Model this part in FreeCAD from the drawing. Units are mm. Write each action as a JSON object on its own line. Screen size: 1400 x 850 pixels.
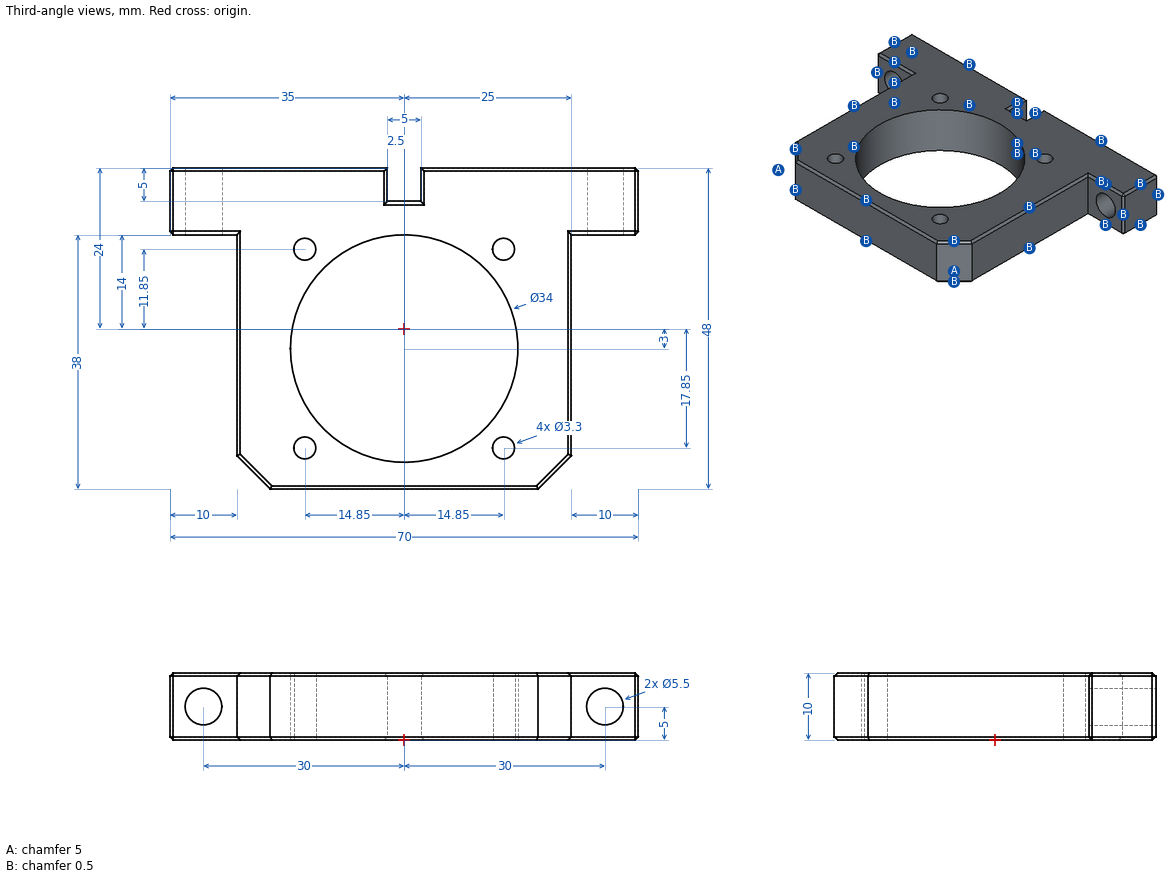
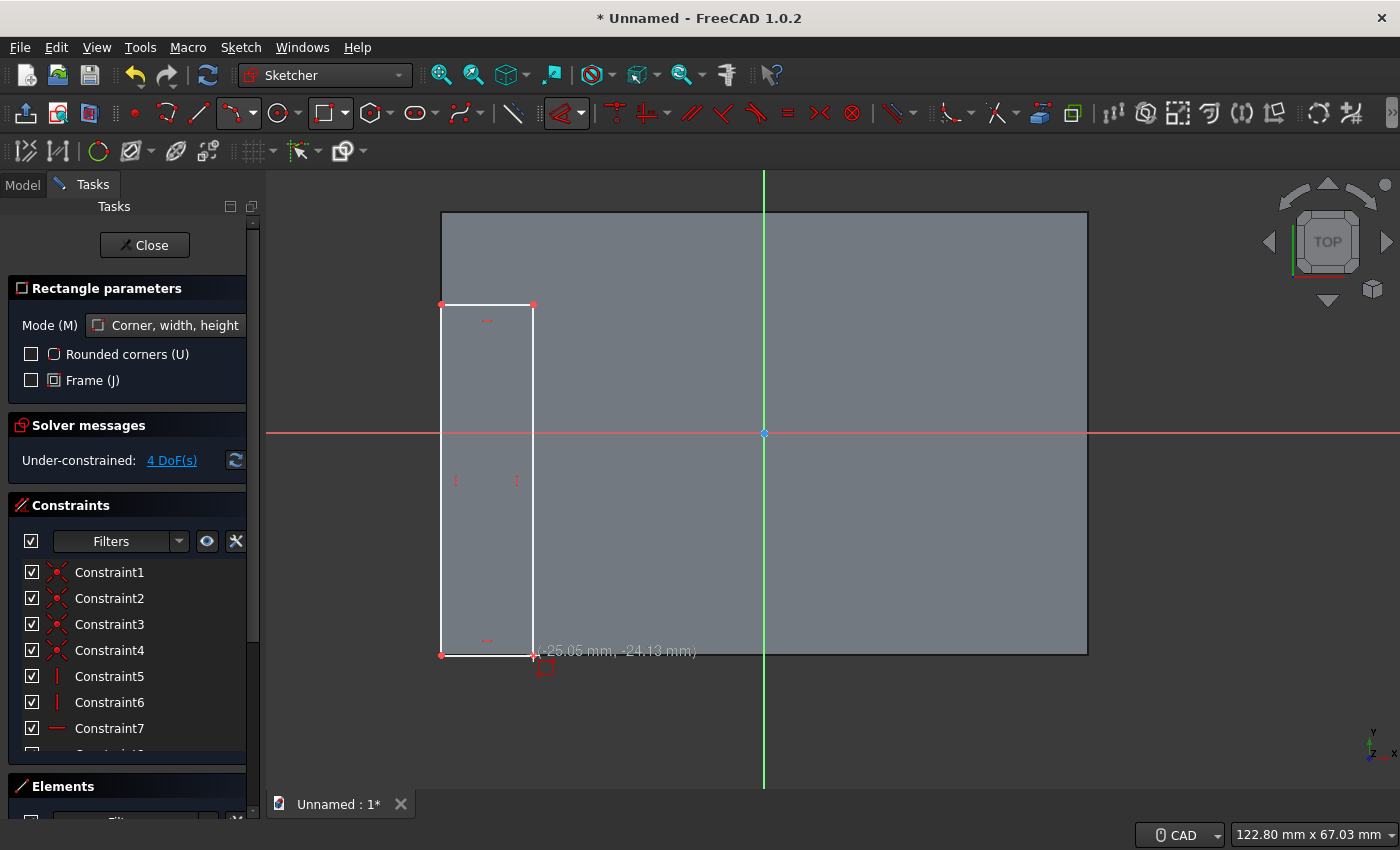
{"action": "left_click", "coordinate": [995, 304]}
{"action": "left_click", "coordinate": [1088, 655]}
{"action": "key", "text": "Escape"}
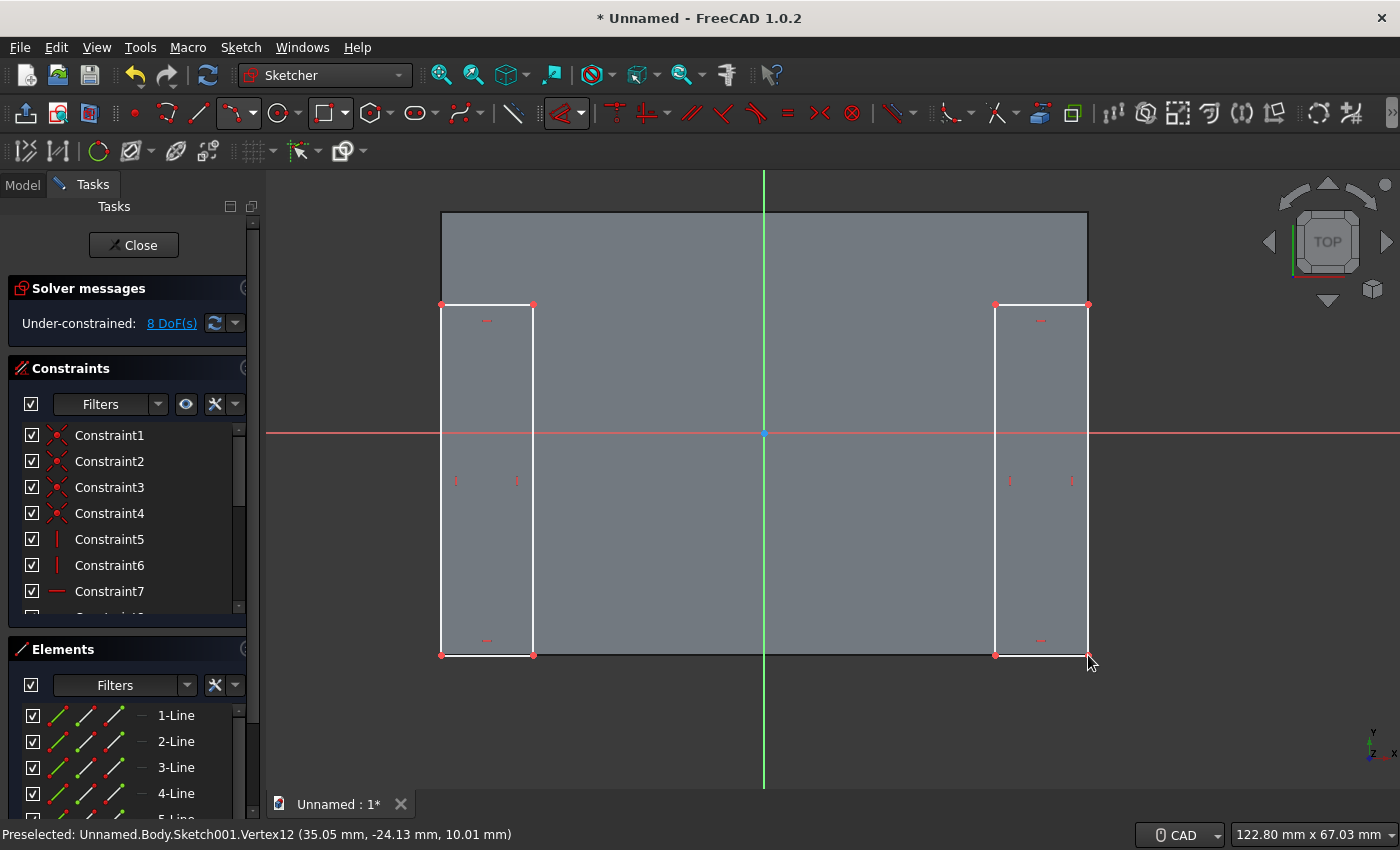
{"action": "left_click", "coordinate": [441, 410]}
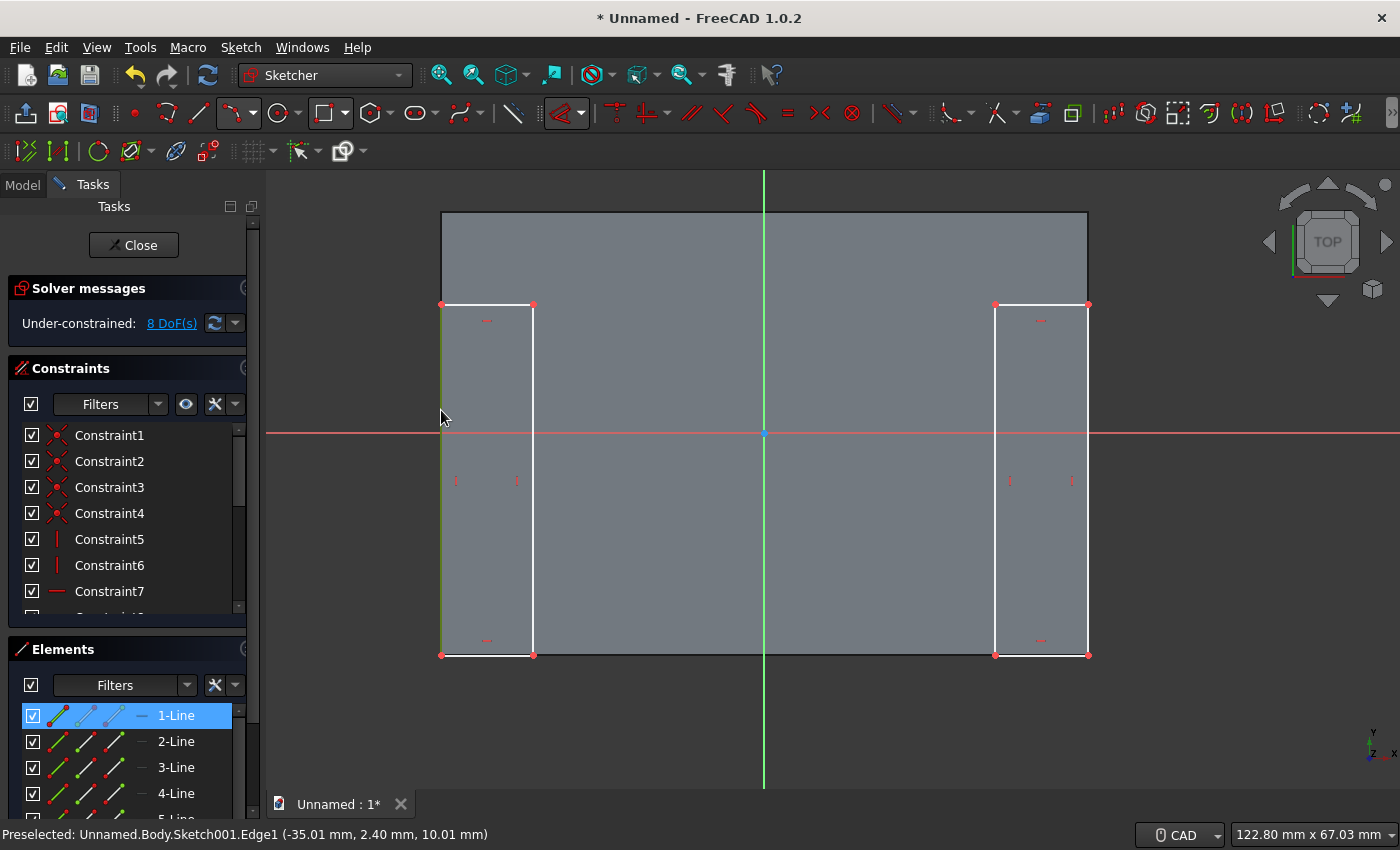
{"action": "key", "text": "i"}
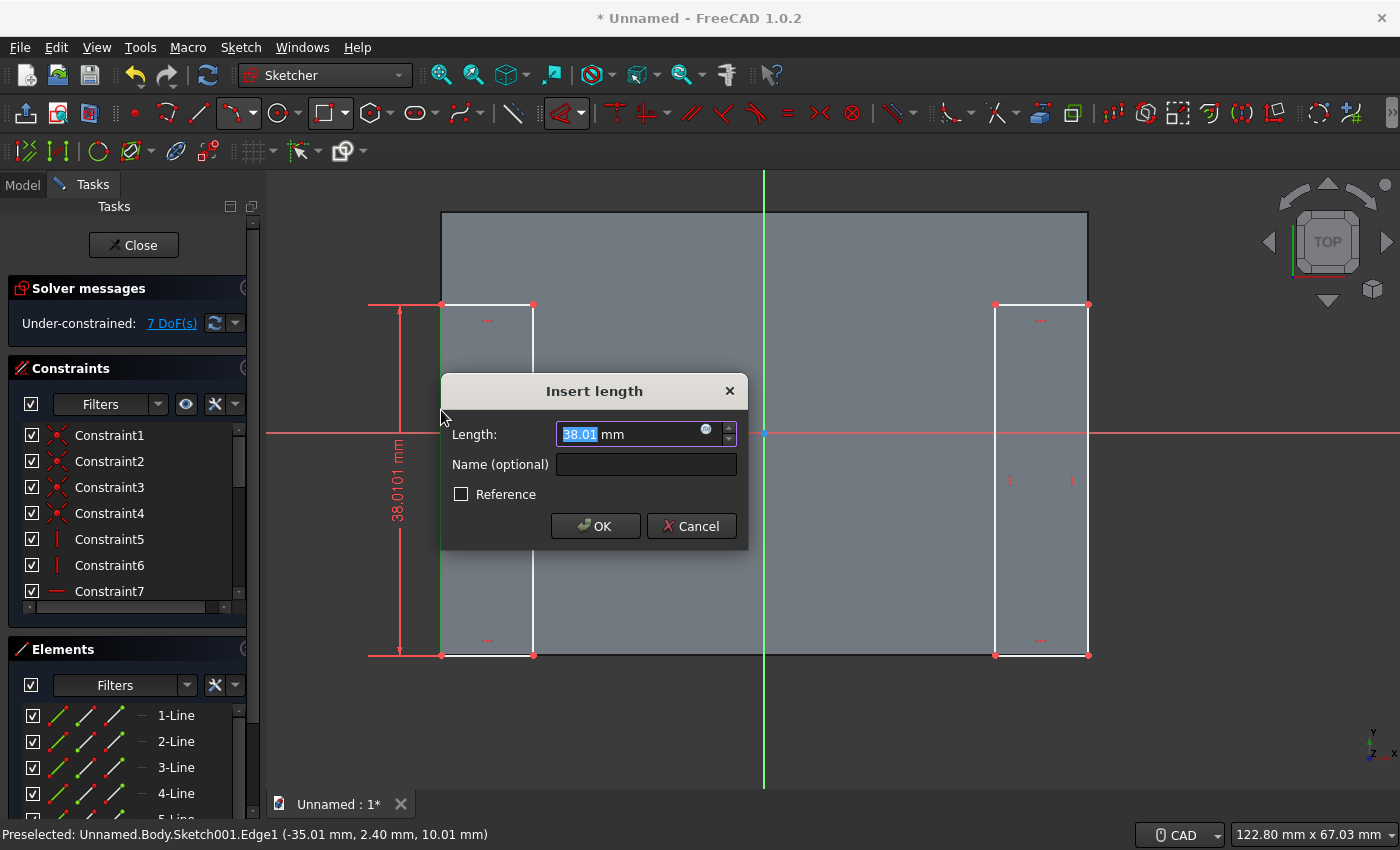
{"action": "type", "text": "38"}
{"action": "key", "text": "Return"}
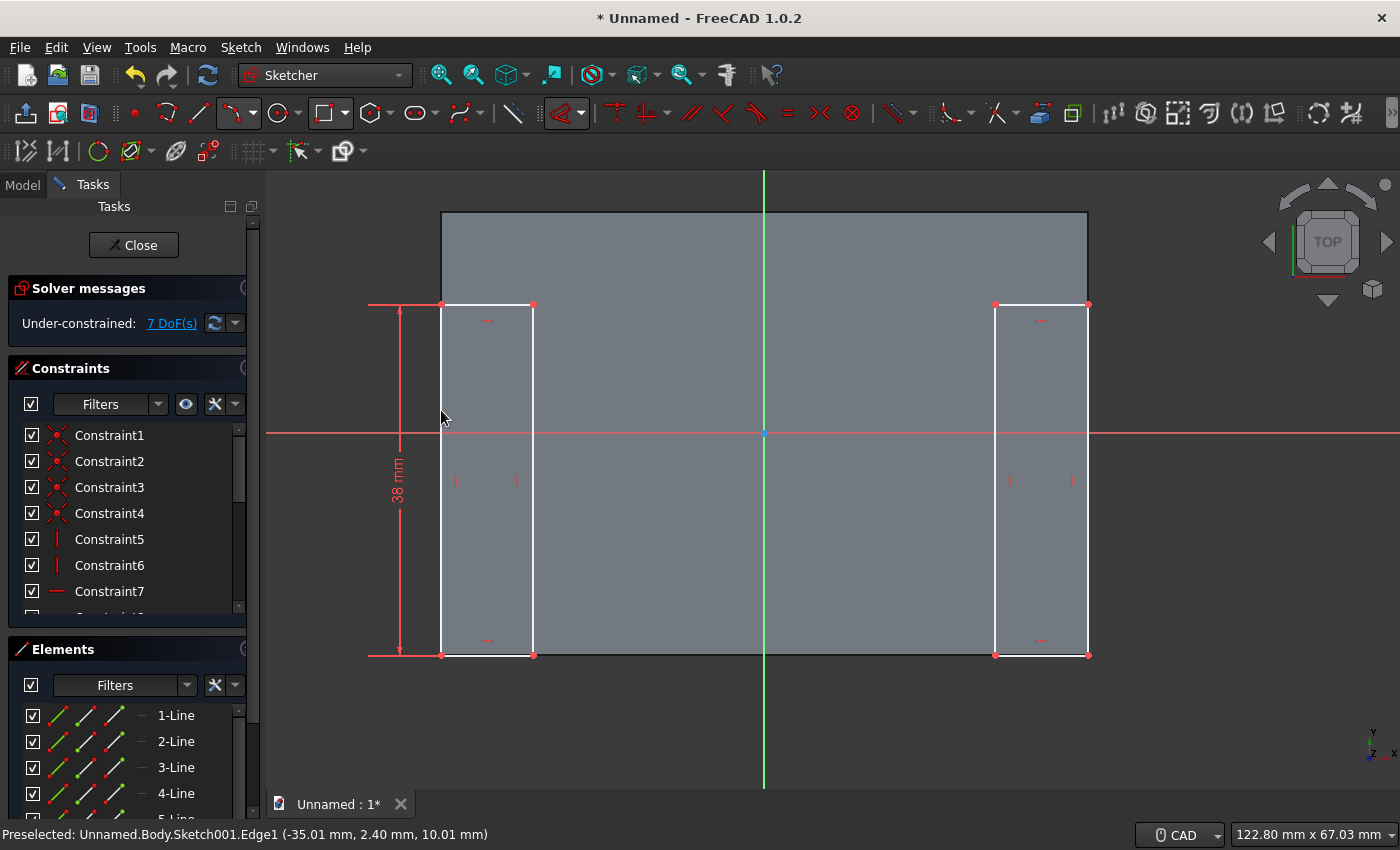
{"action": "left_click", "coordinate": [469, 656]}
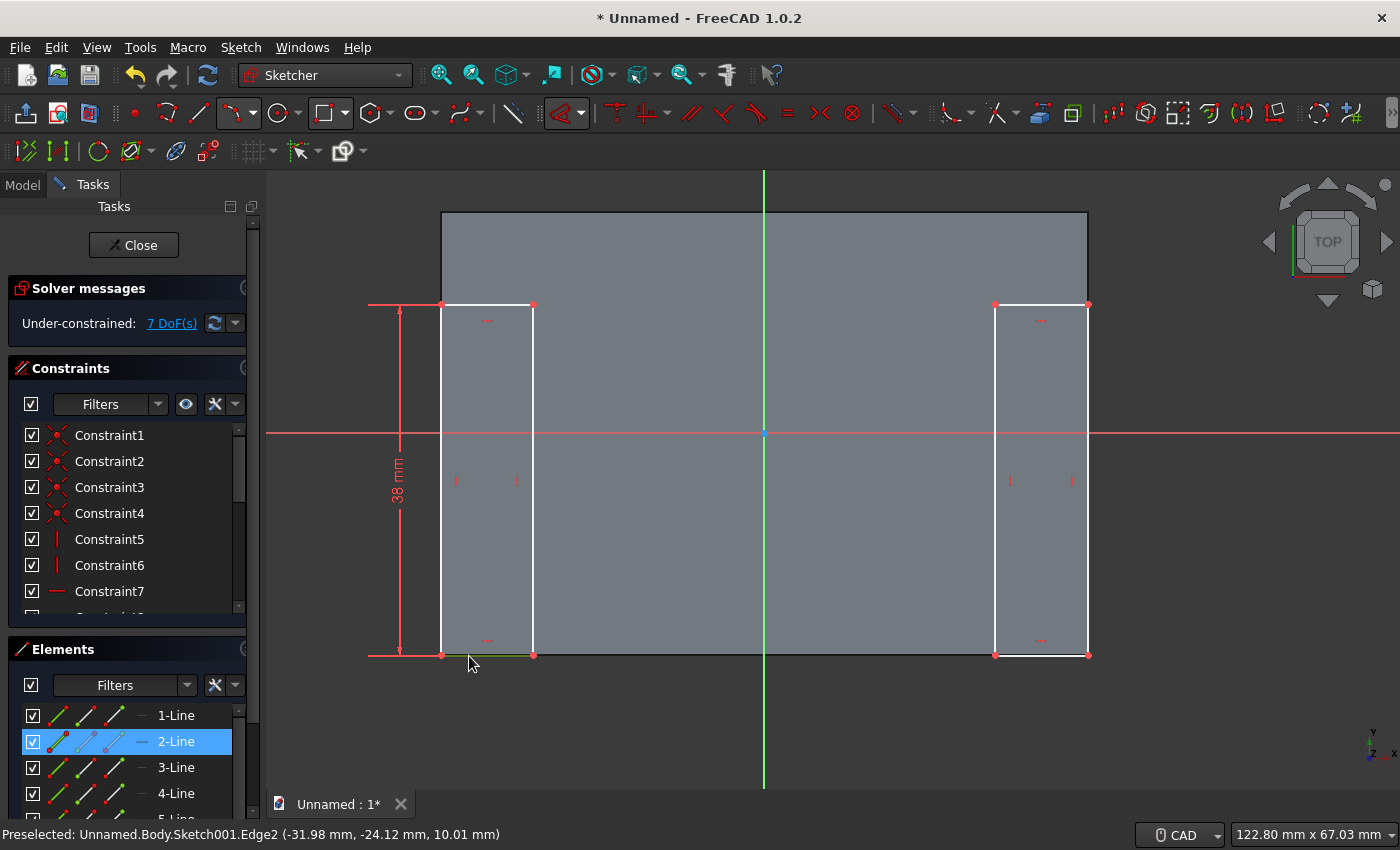
{"action": "left_click", "coordinate": [584, 114]}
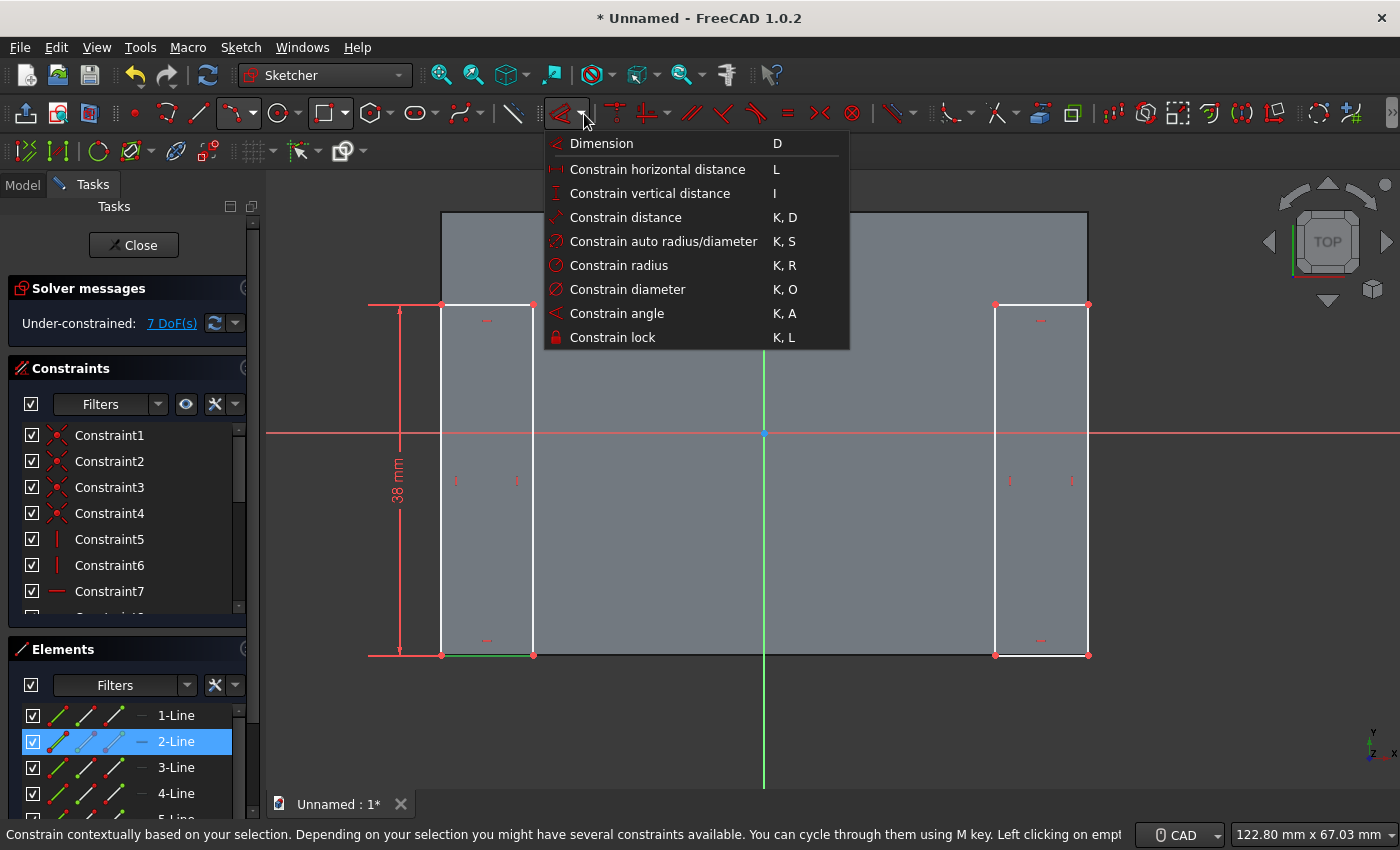
{"action": "left_click", "coordinate": [697, 169]}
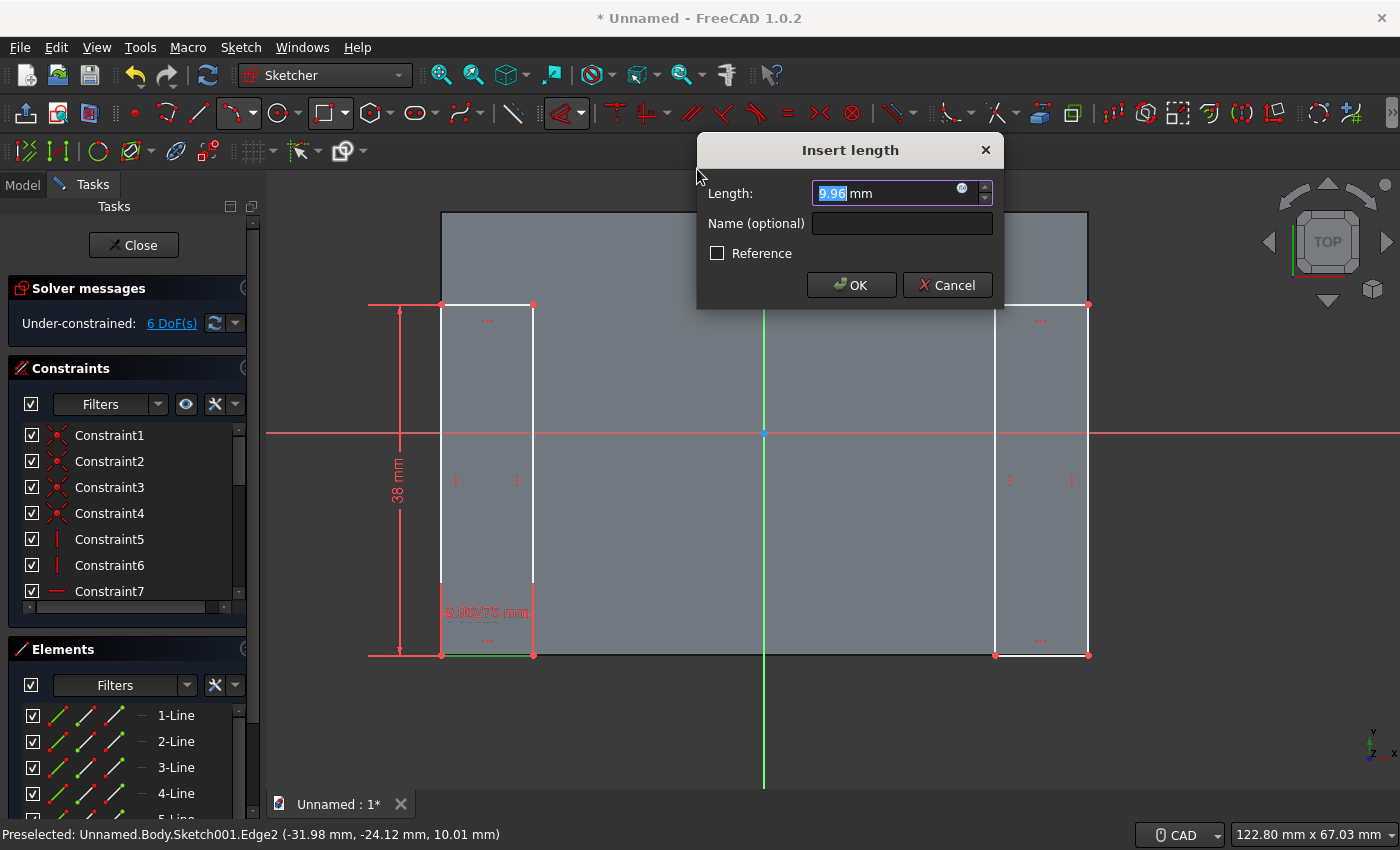
{"action": "type", "text": "10"}
{"action": "key", "text": "Return"}